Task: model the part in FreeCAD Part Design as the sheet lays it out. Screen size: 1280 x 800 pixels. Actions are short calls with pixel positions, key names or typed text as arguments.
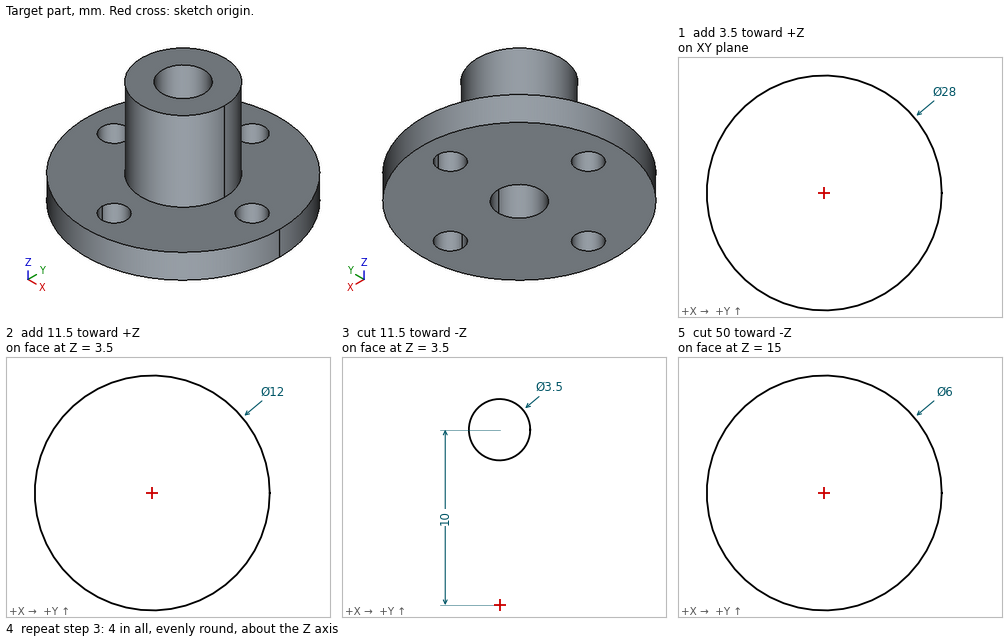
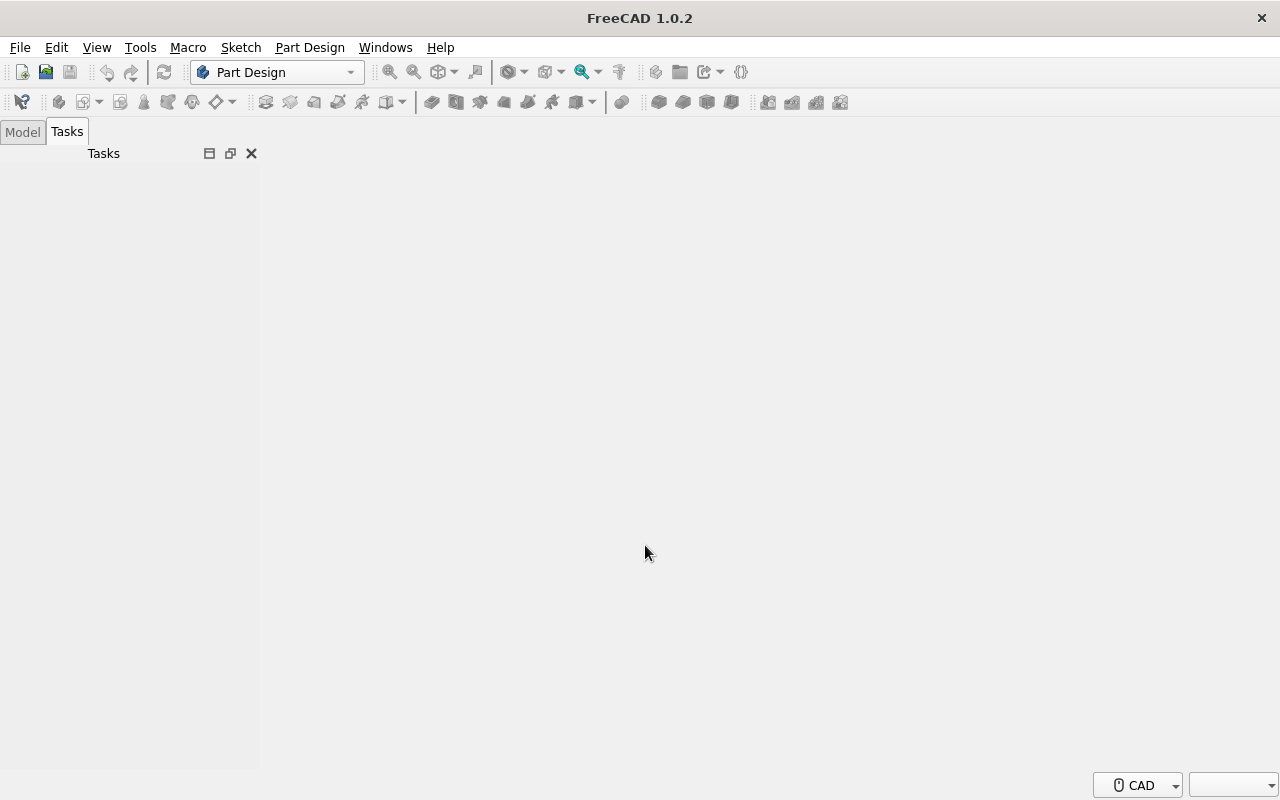
key(ctrl+n)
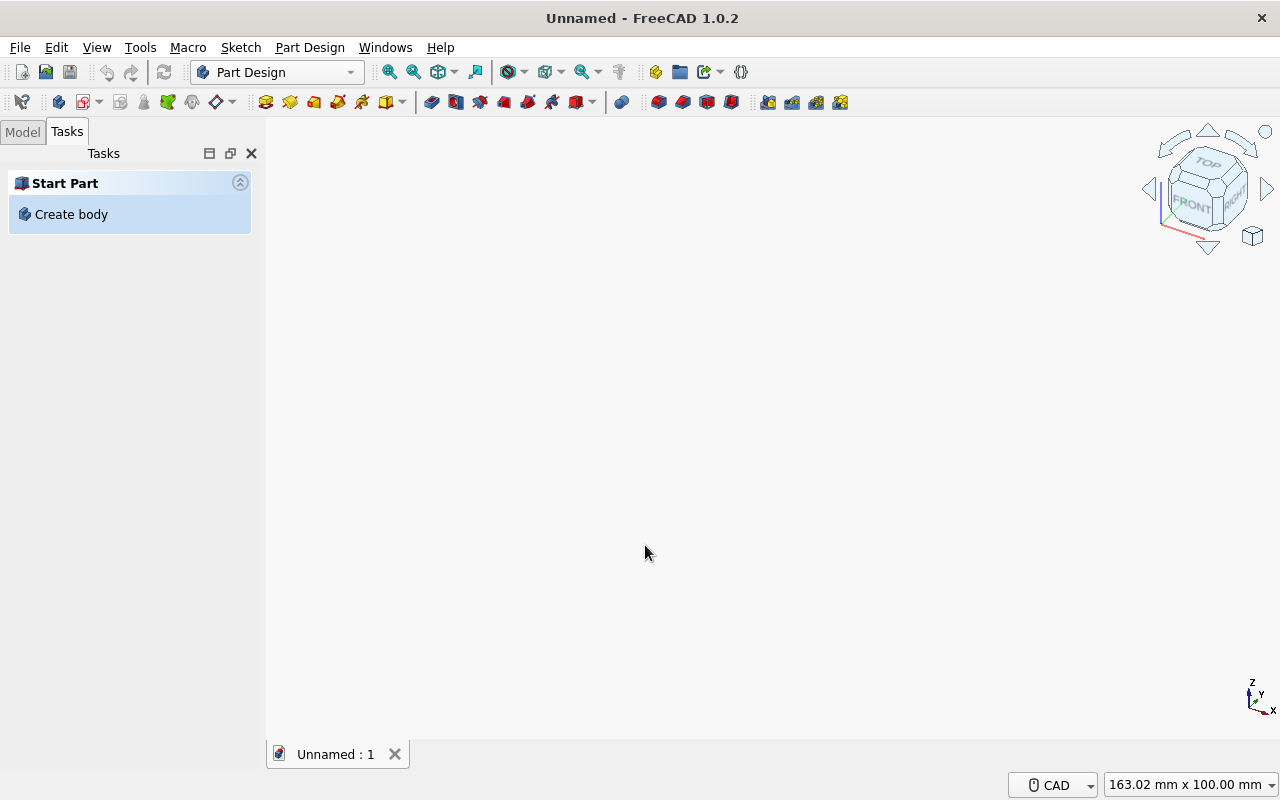
click(84, 102)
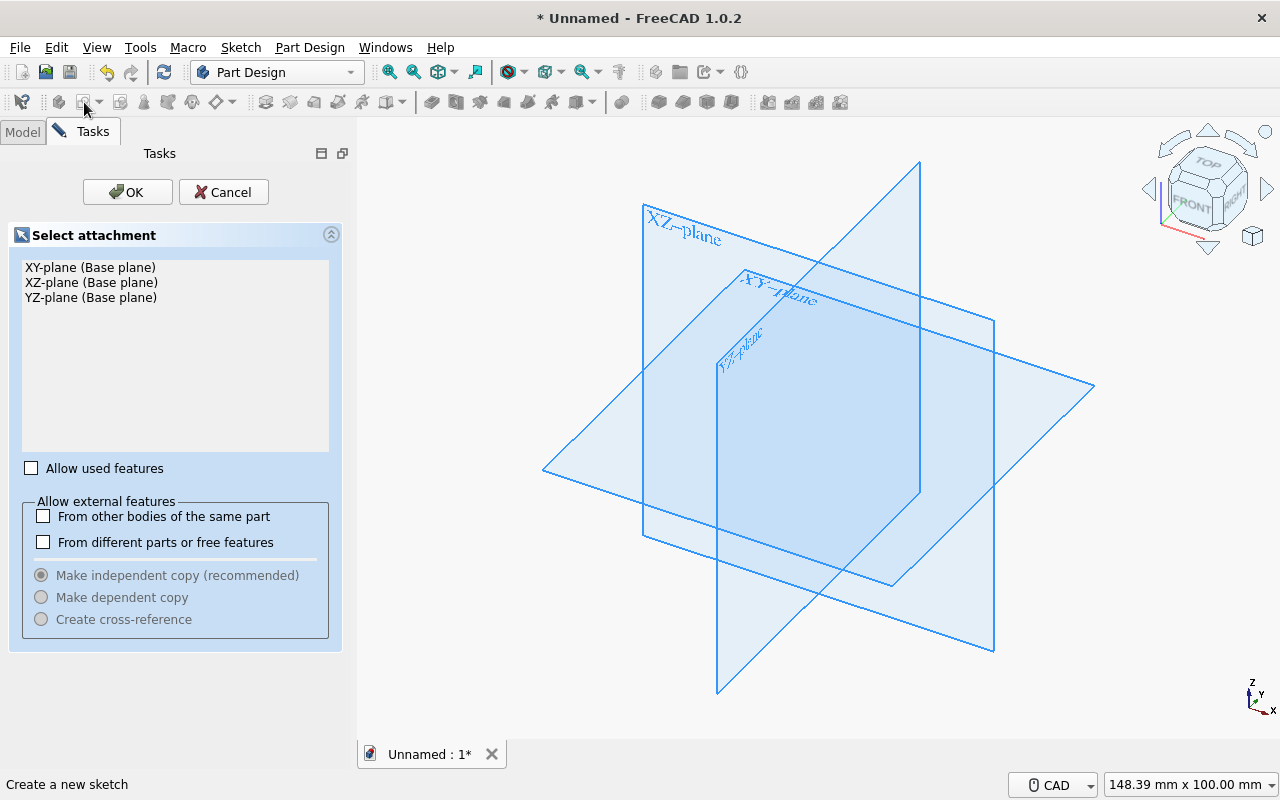
click(82, 268)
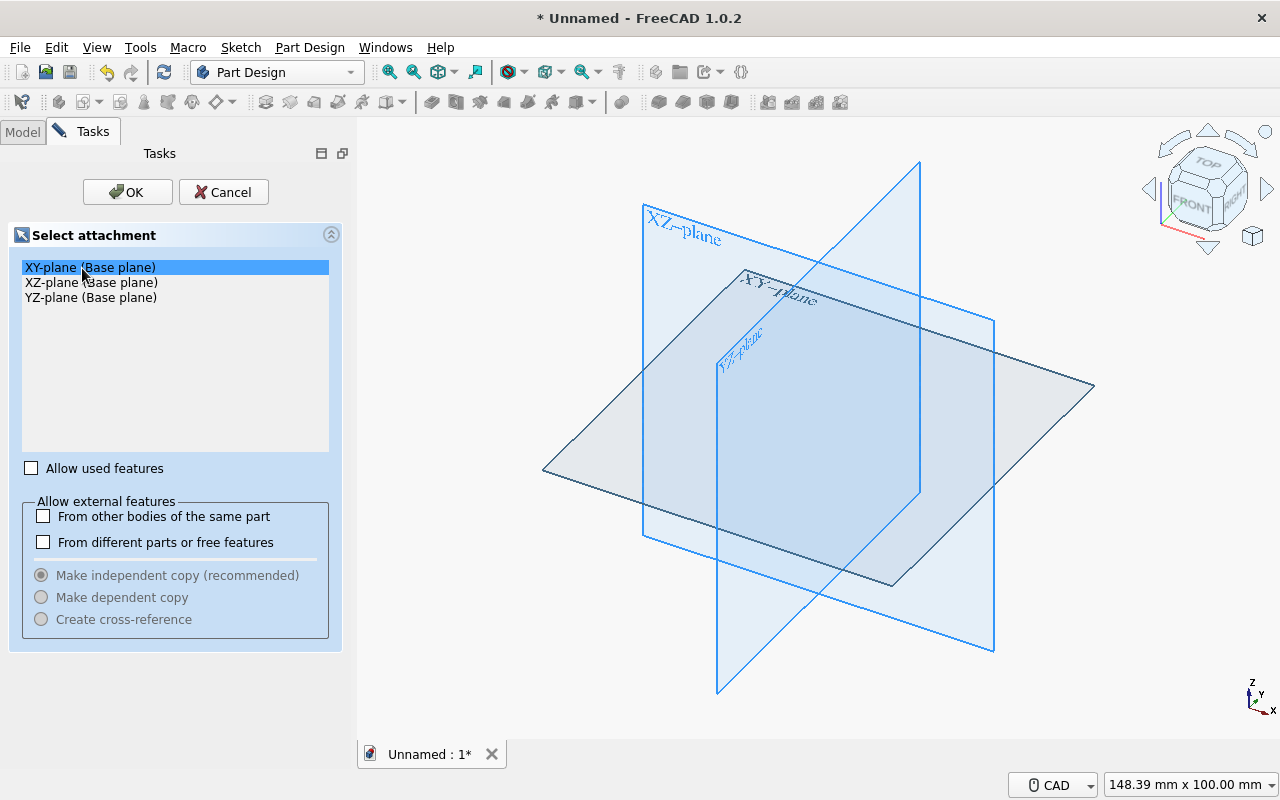
click(128, 192)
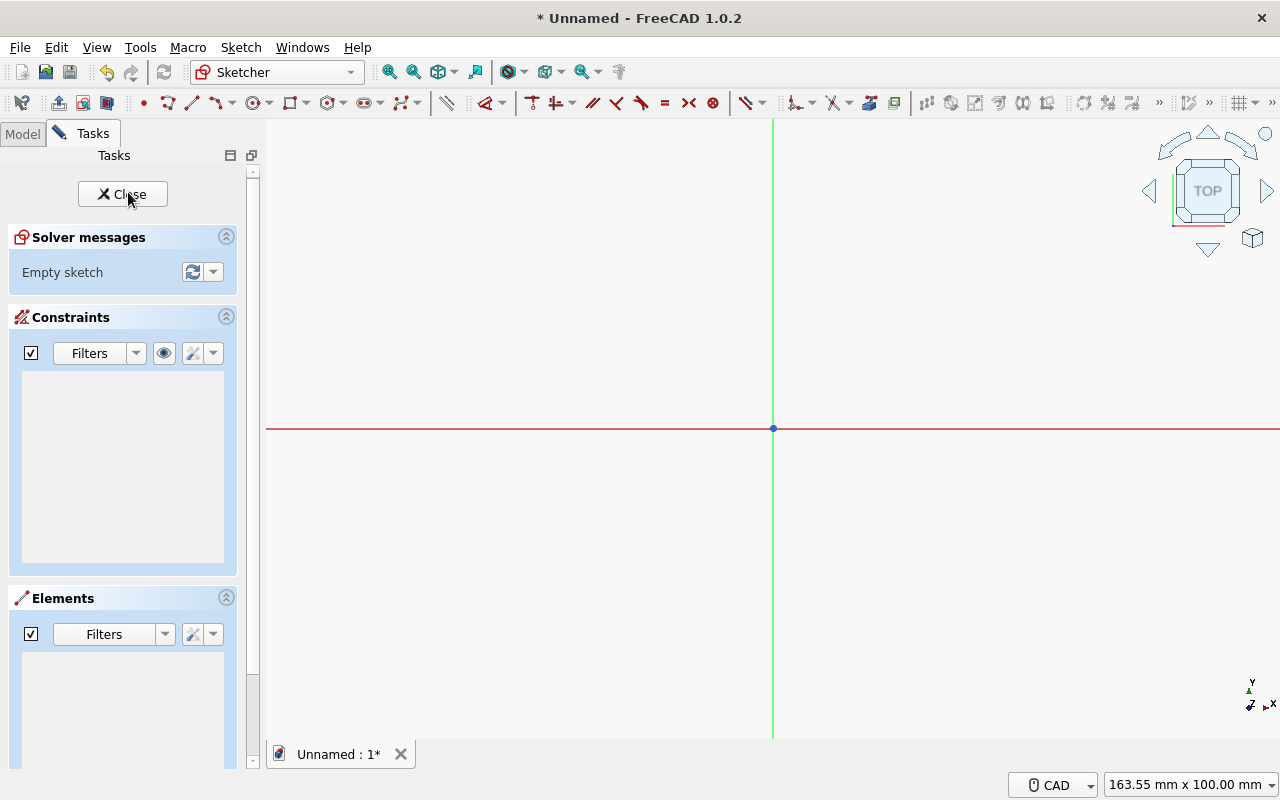
scroll(829, 429, up, 4)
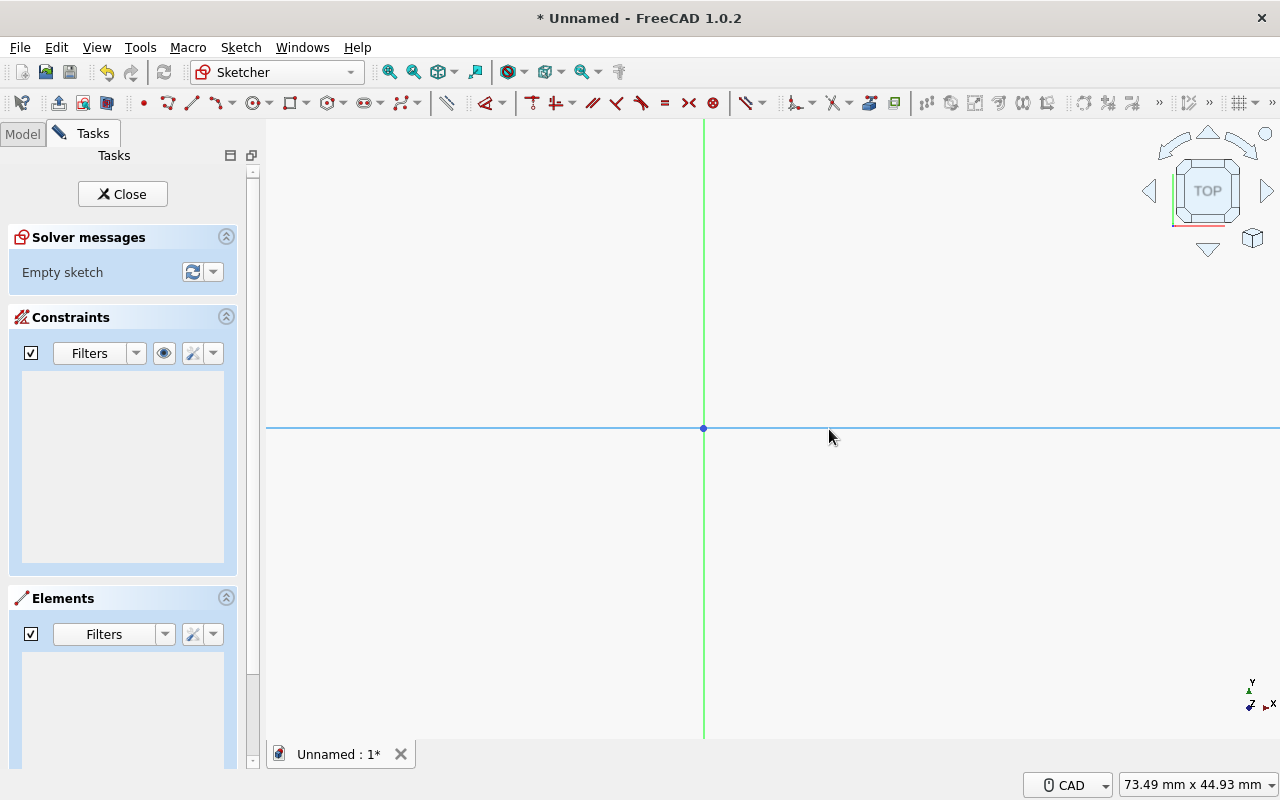
key(g)
key(c)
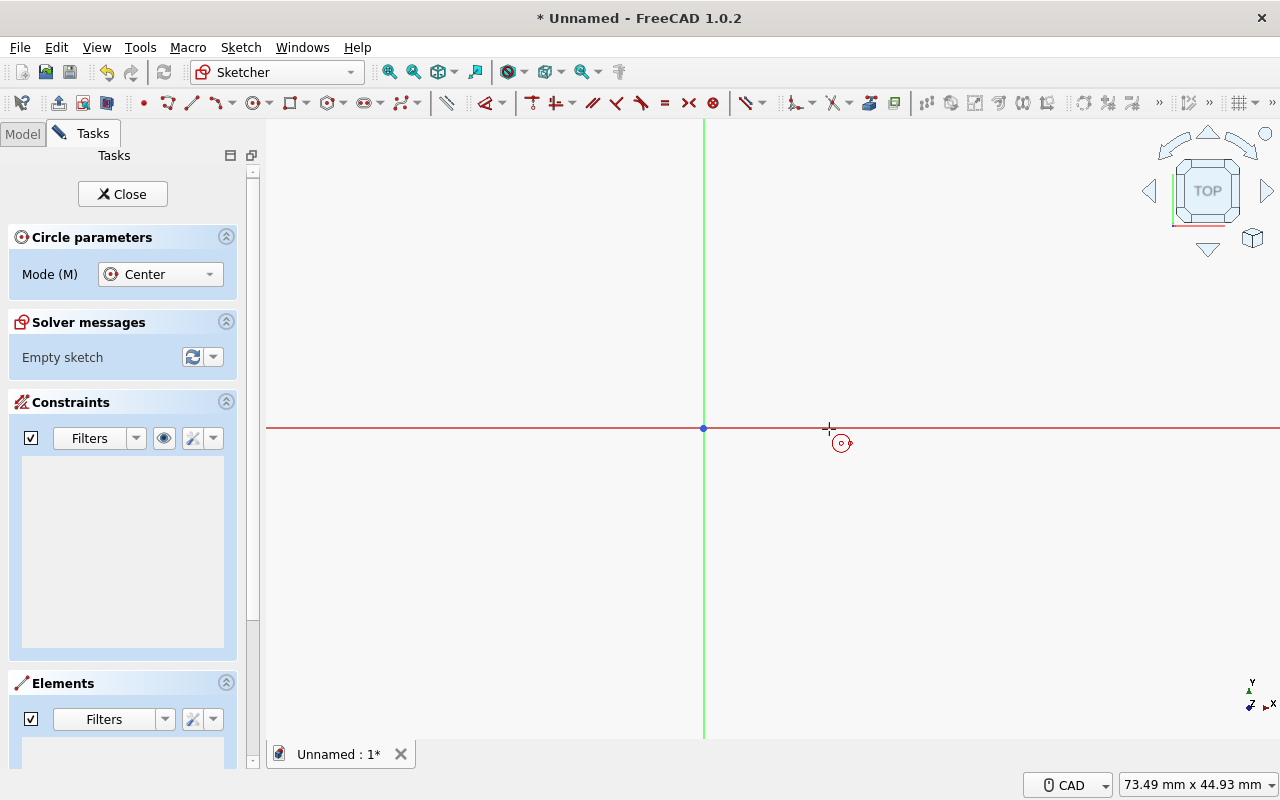
click(704, 428)
click(840, 292)
key(Escape)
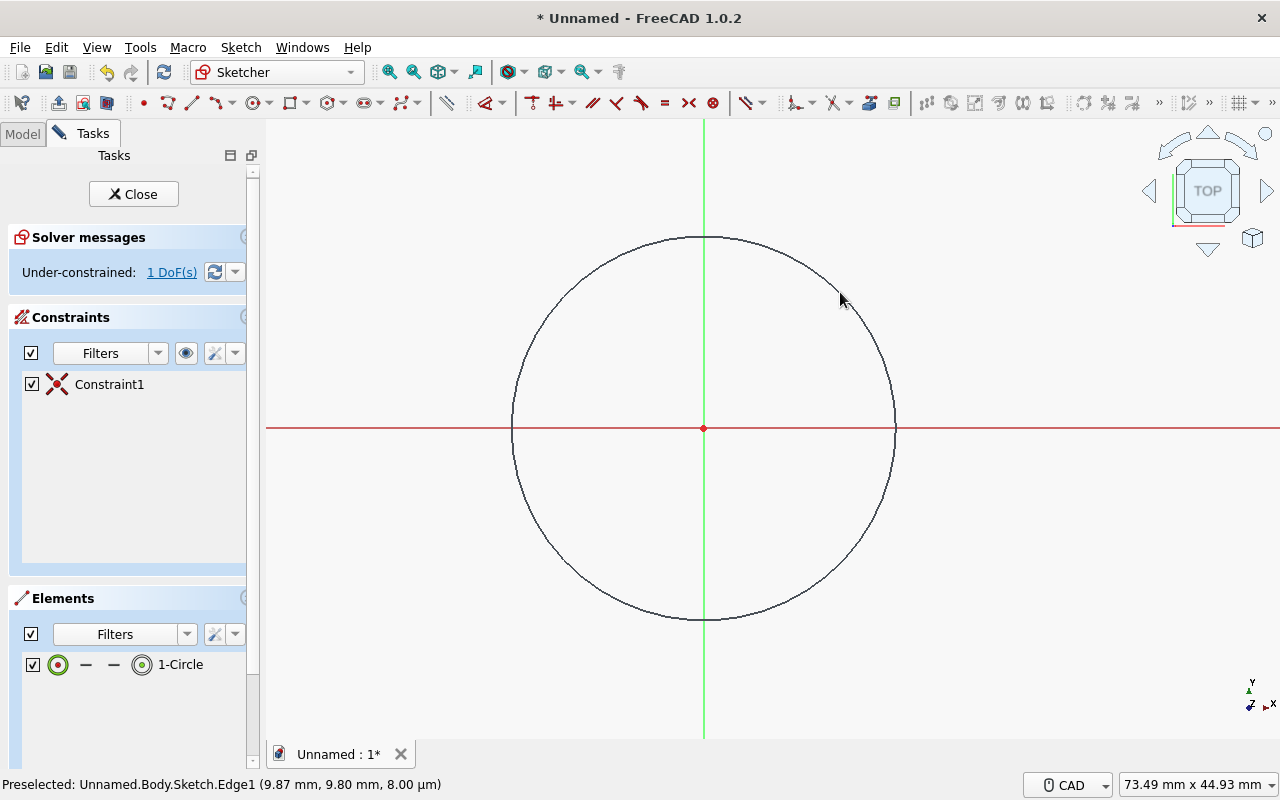
click(486, 104)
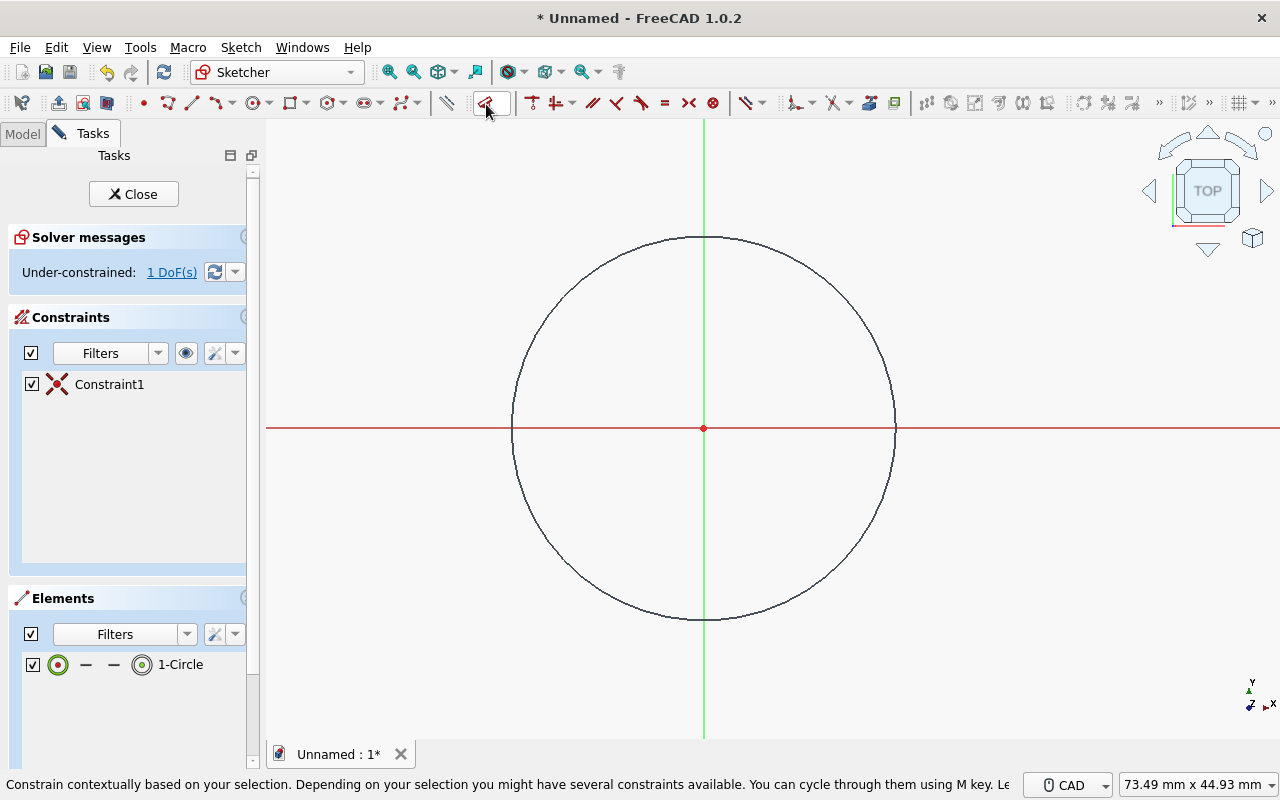
click(839, 292)
click(862, 269)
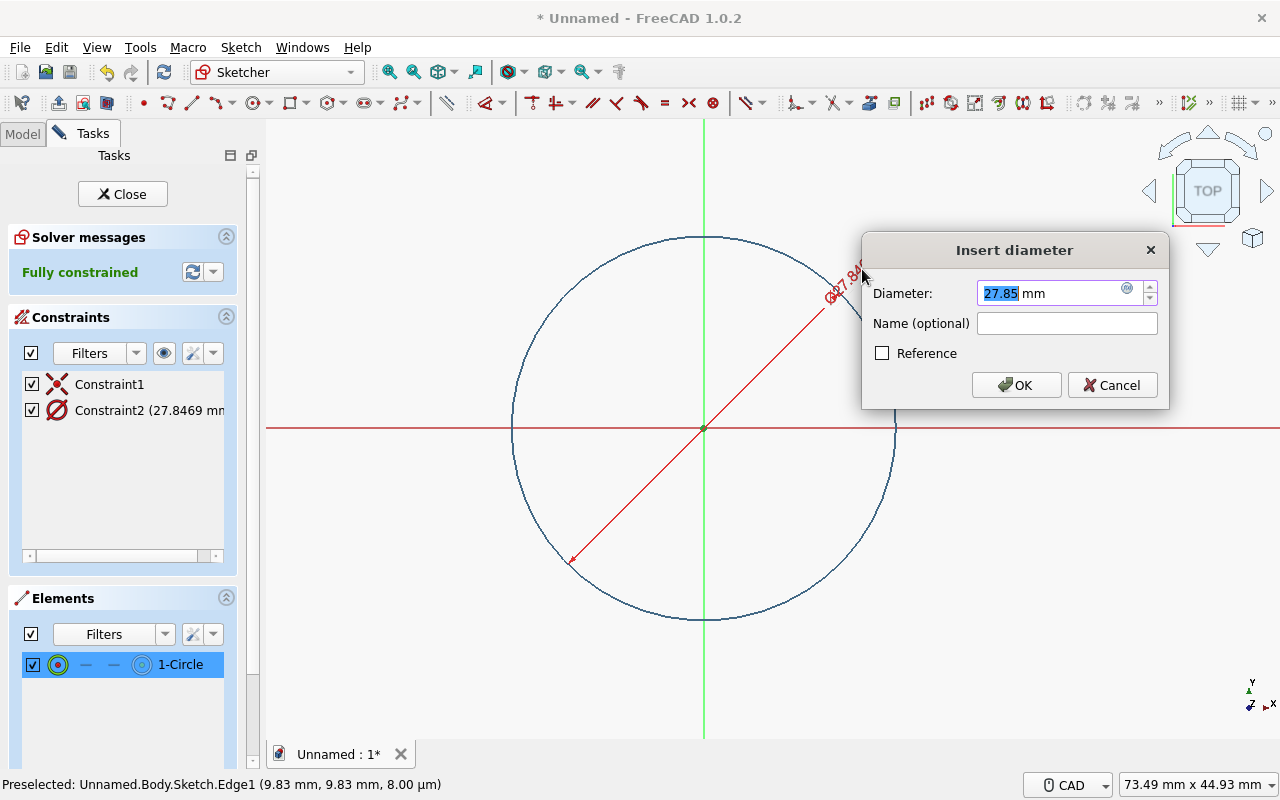
text(28)
key(Return)
key(Escape)